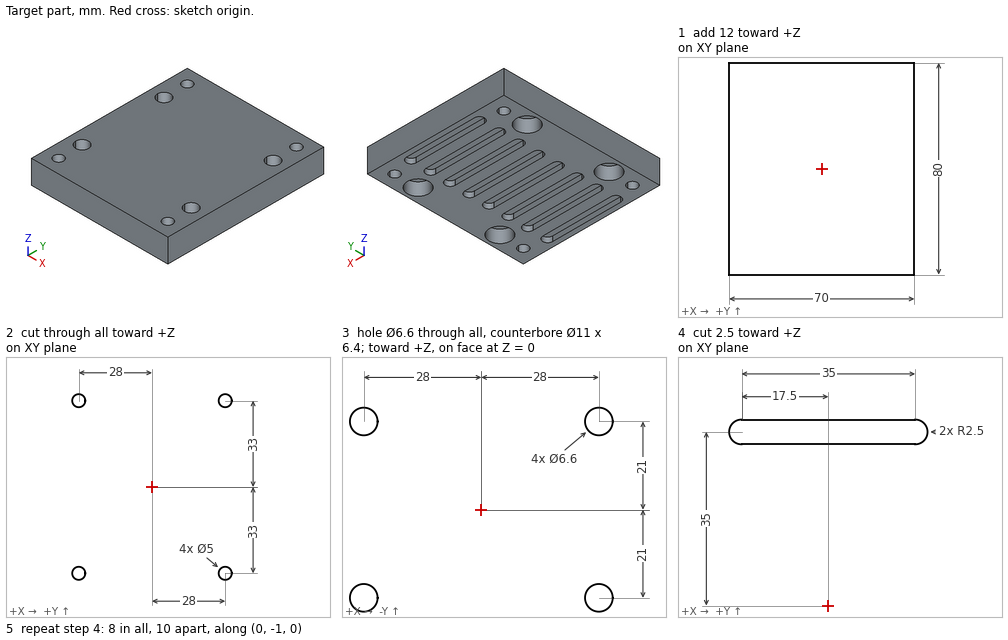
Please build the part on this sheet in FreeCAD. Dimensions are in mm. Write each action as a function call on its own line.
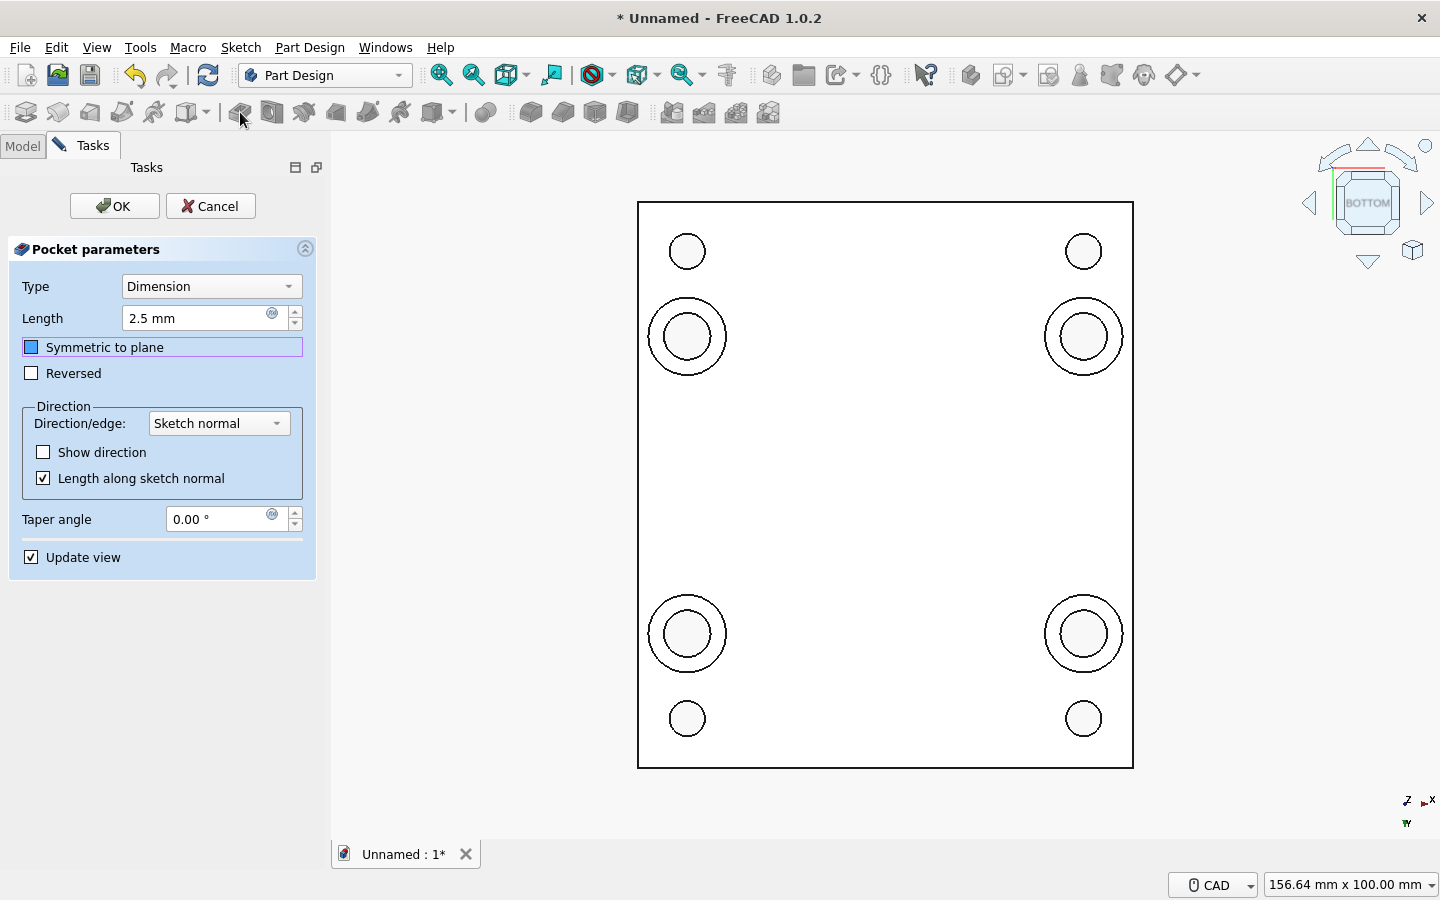
click(30, 373)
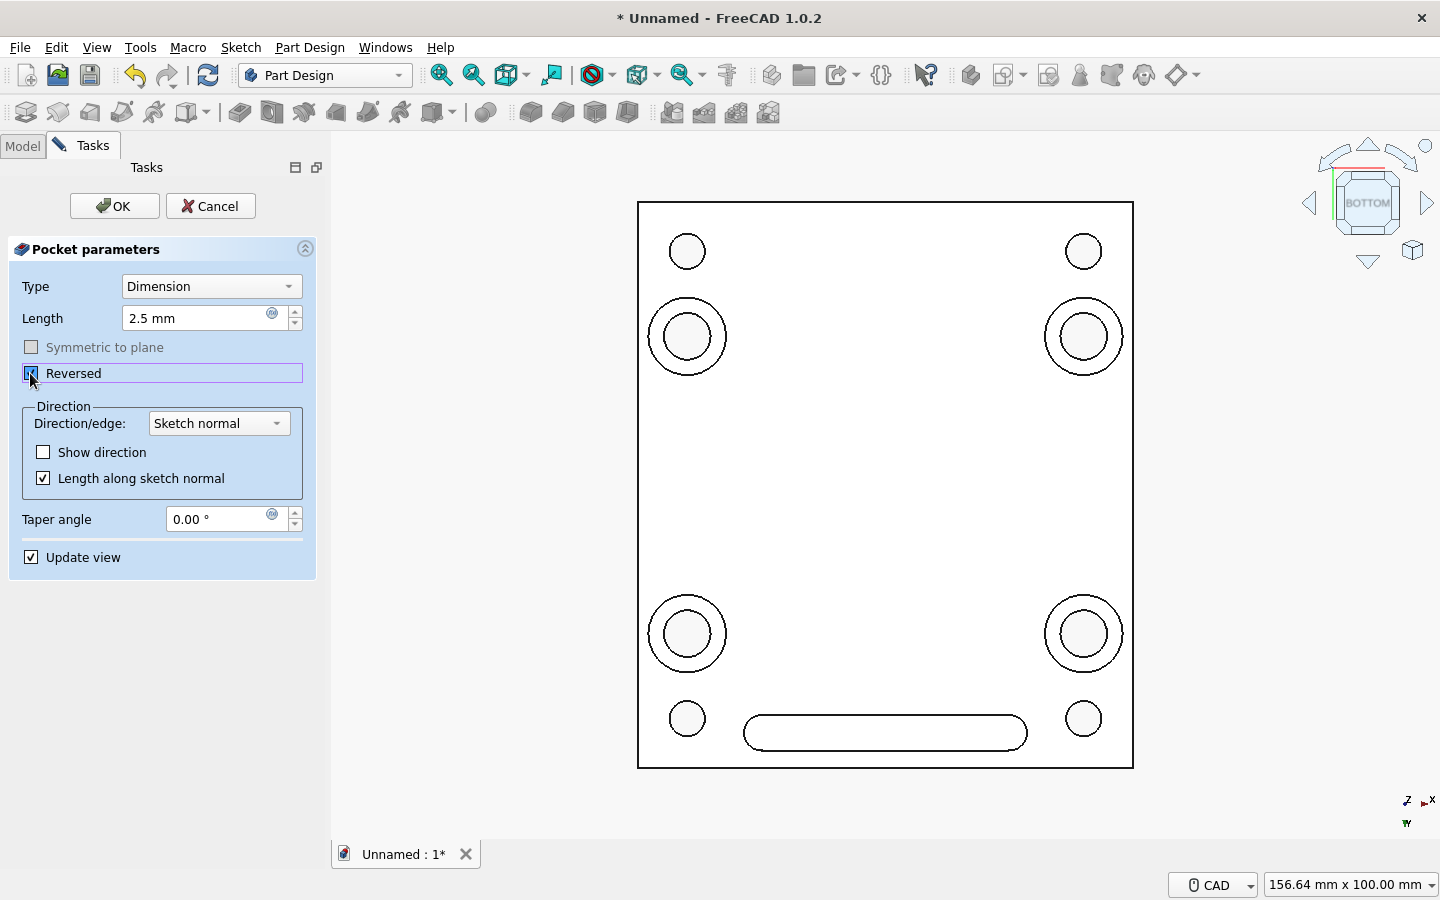
click(115, 206)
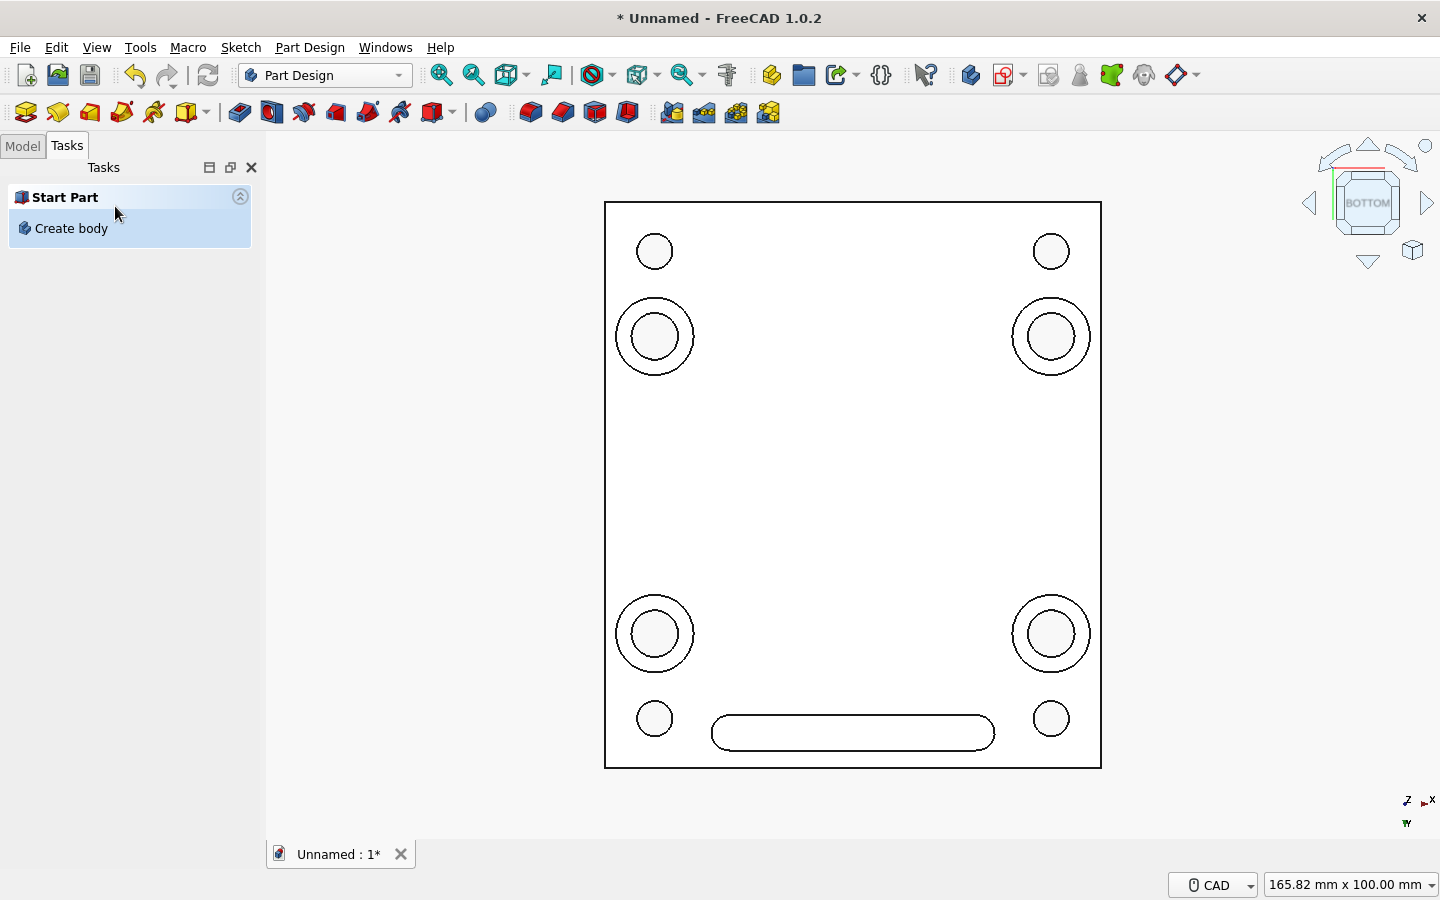
click(23, 145)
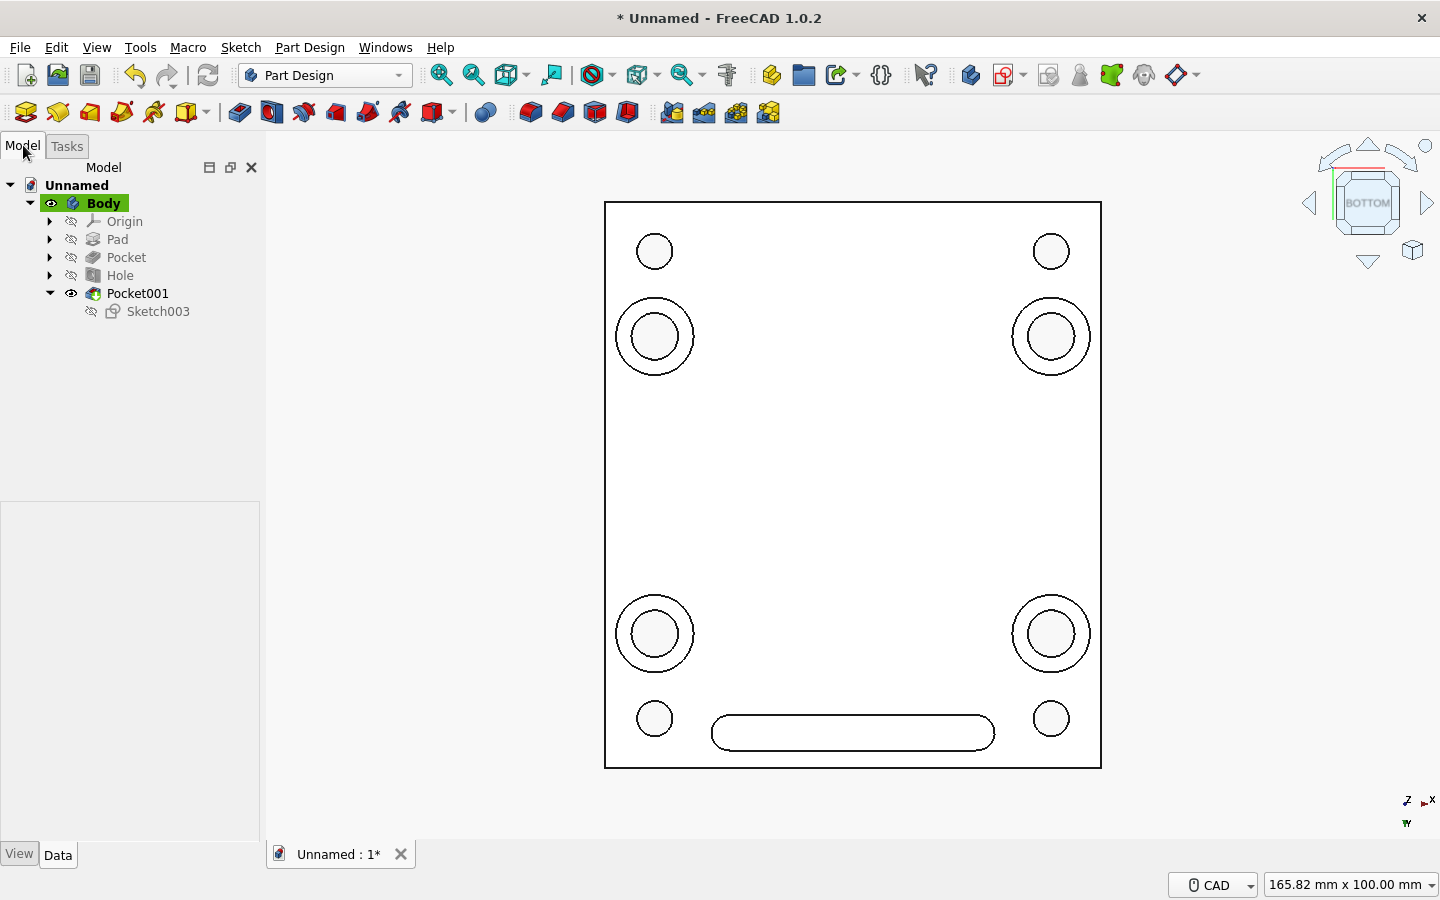
click(116, 293)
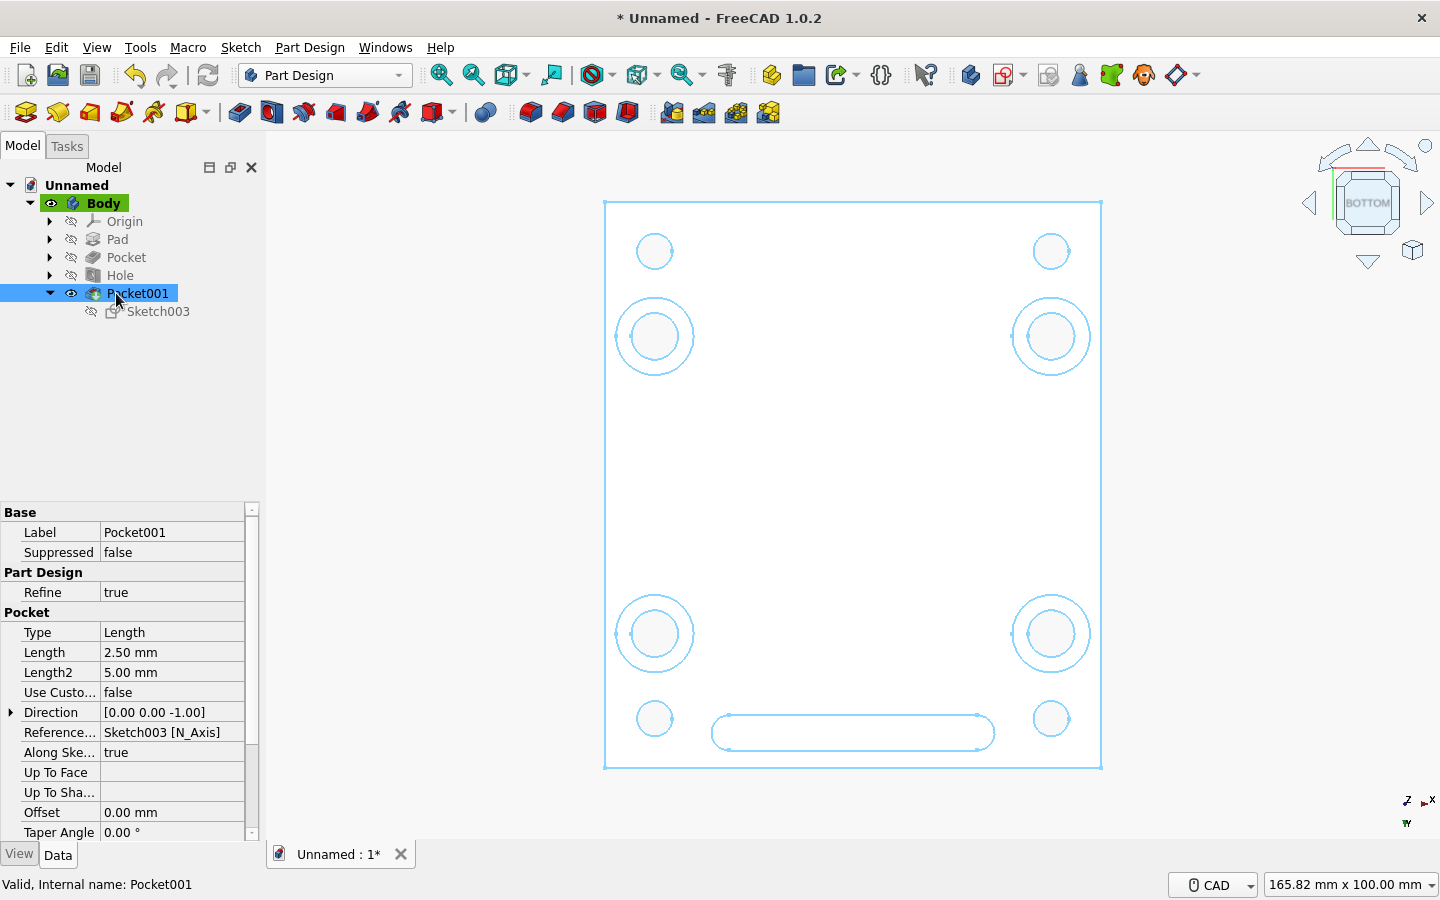
click(704, 112)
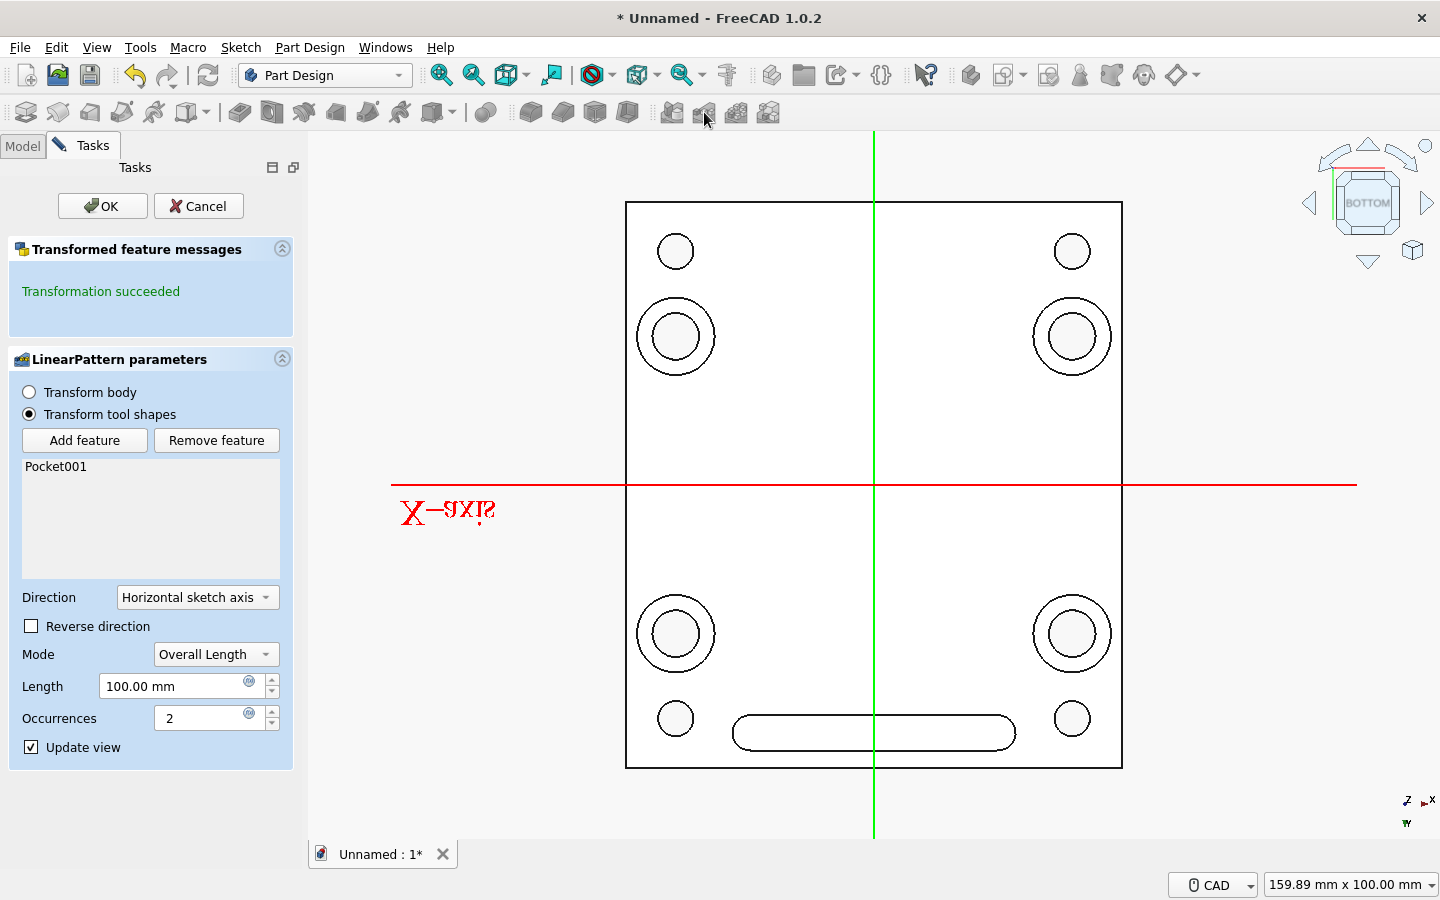
click(198, 598)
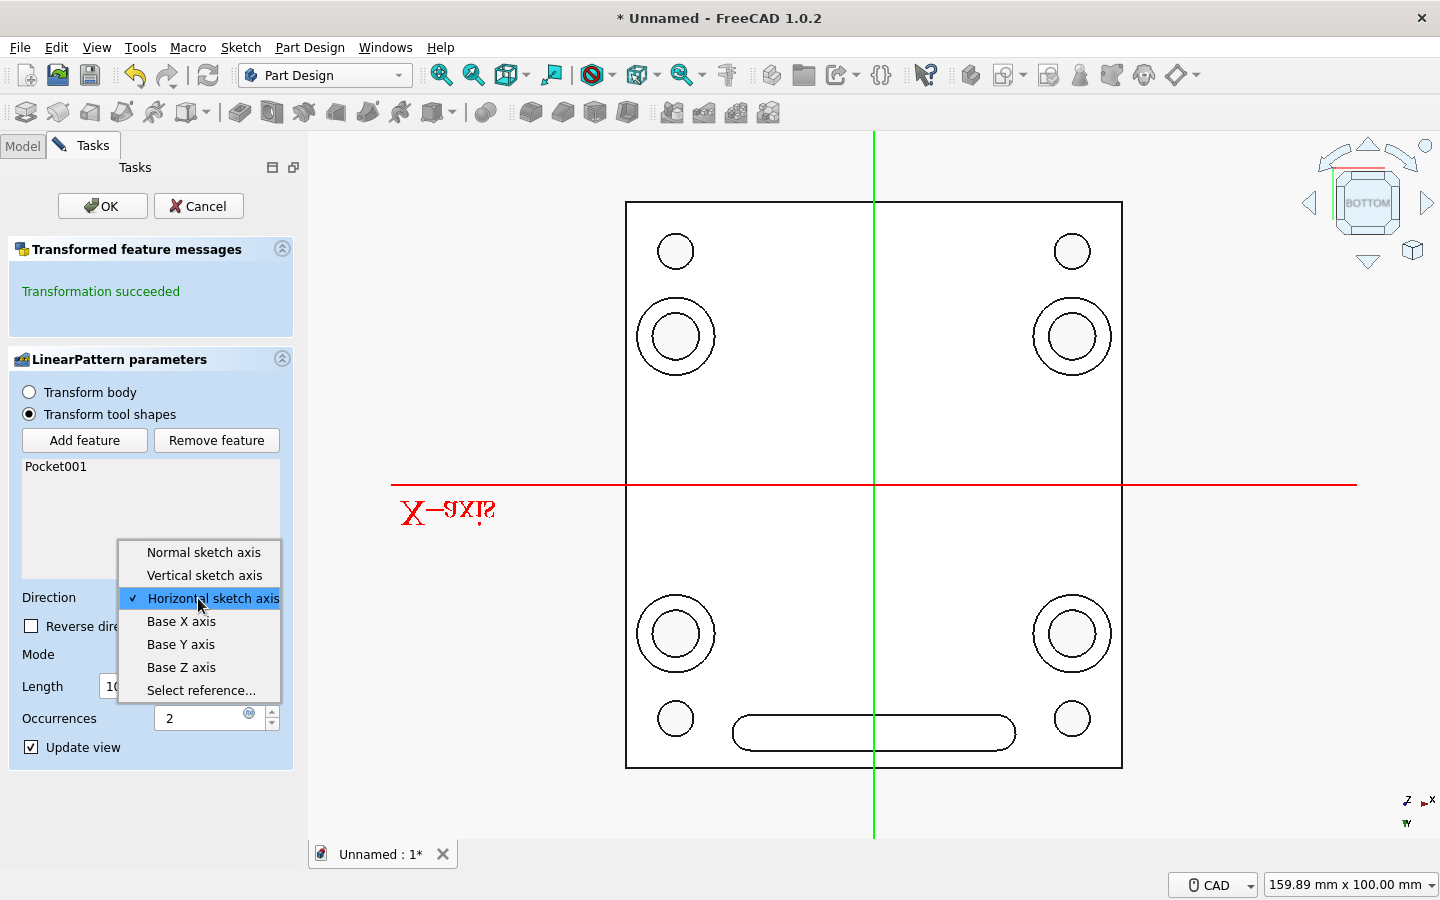
click(198, 644)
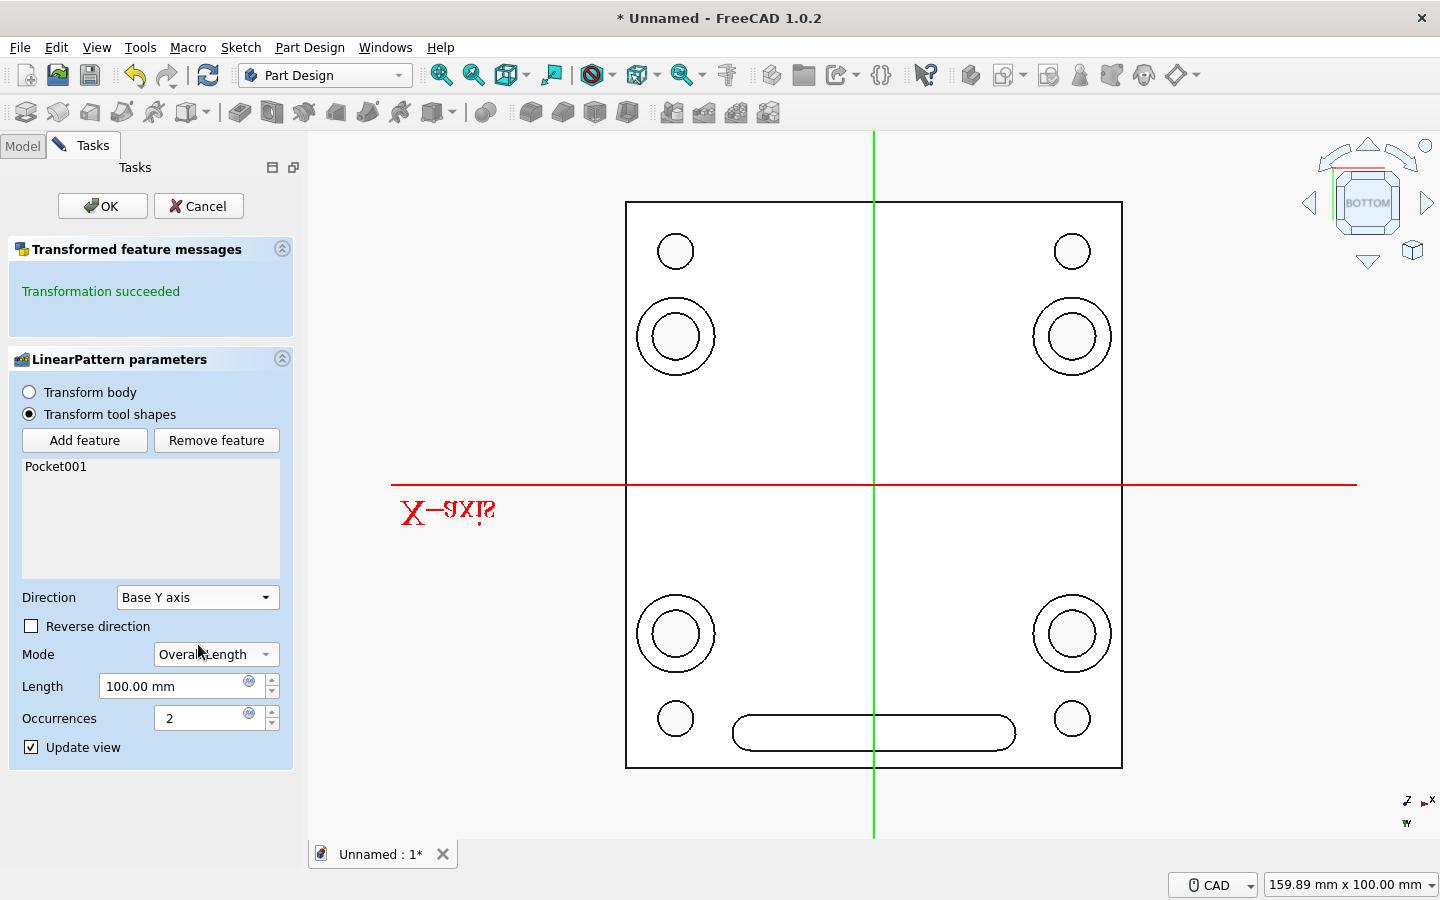
click(217, 654)